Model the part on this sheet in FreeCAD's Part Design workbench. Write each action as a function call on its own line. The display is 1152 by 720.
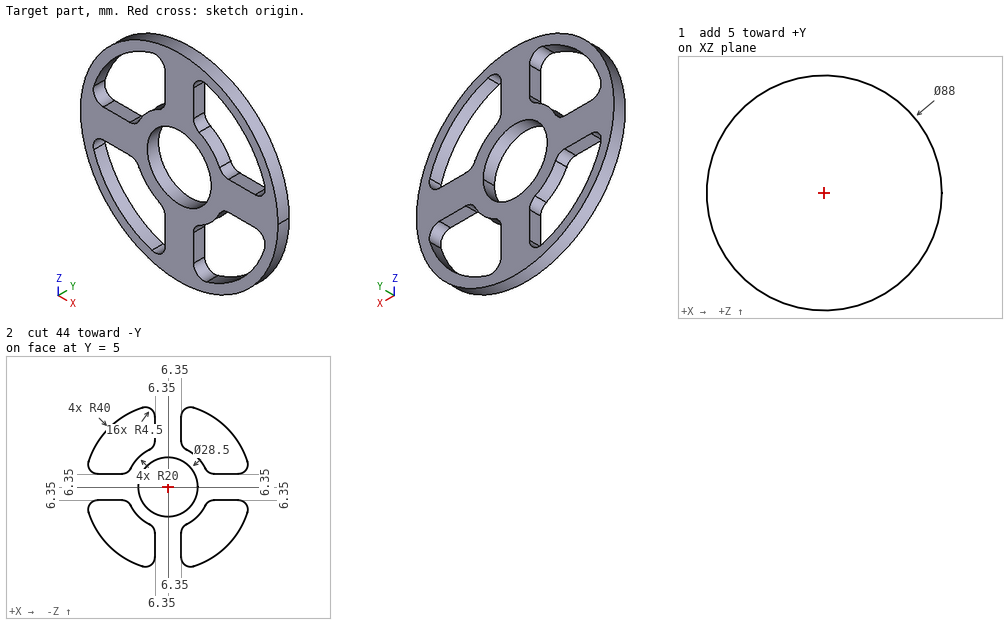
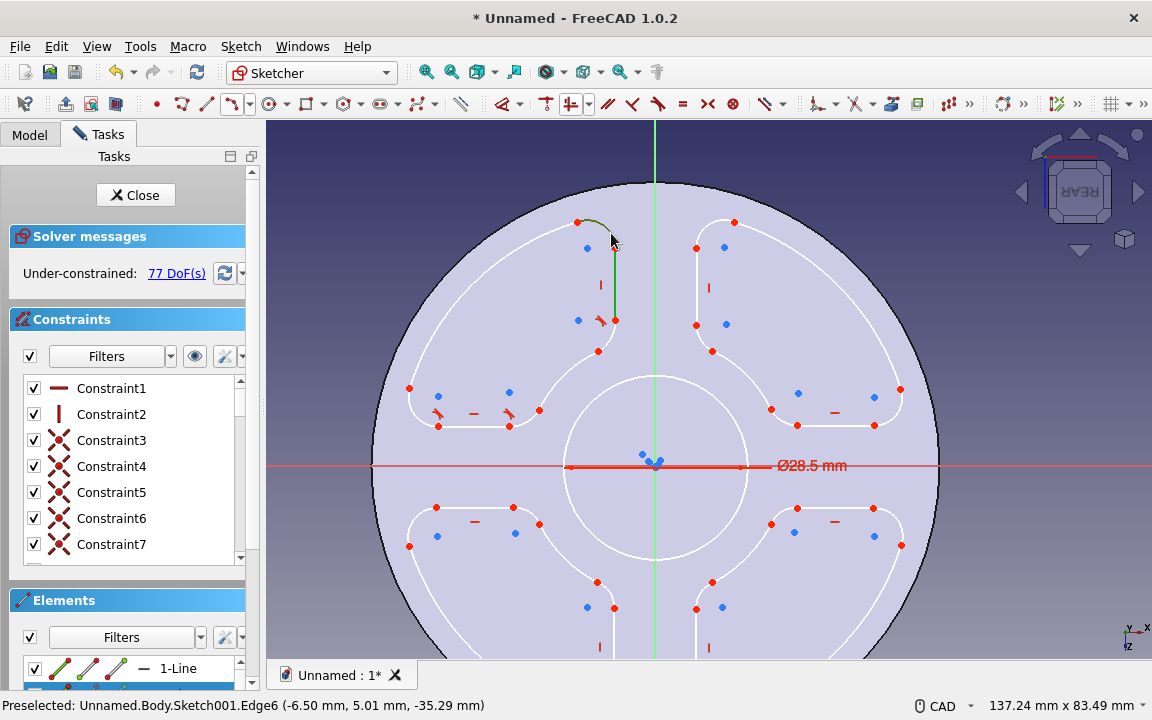
key(t)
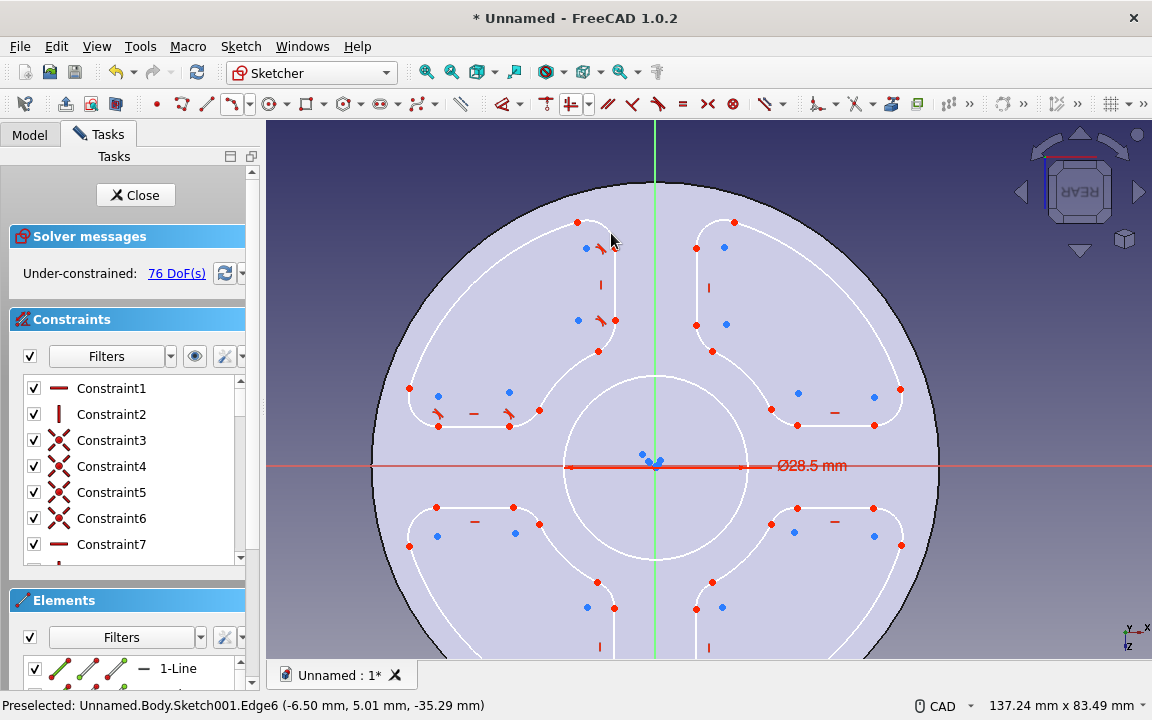
scroll(520, 425, up, 2)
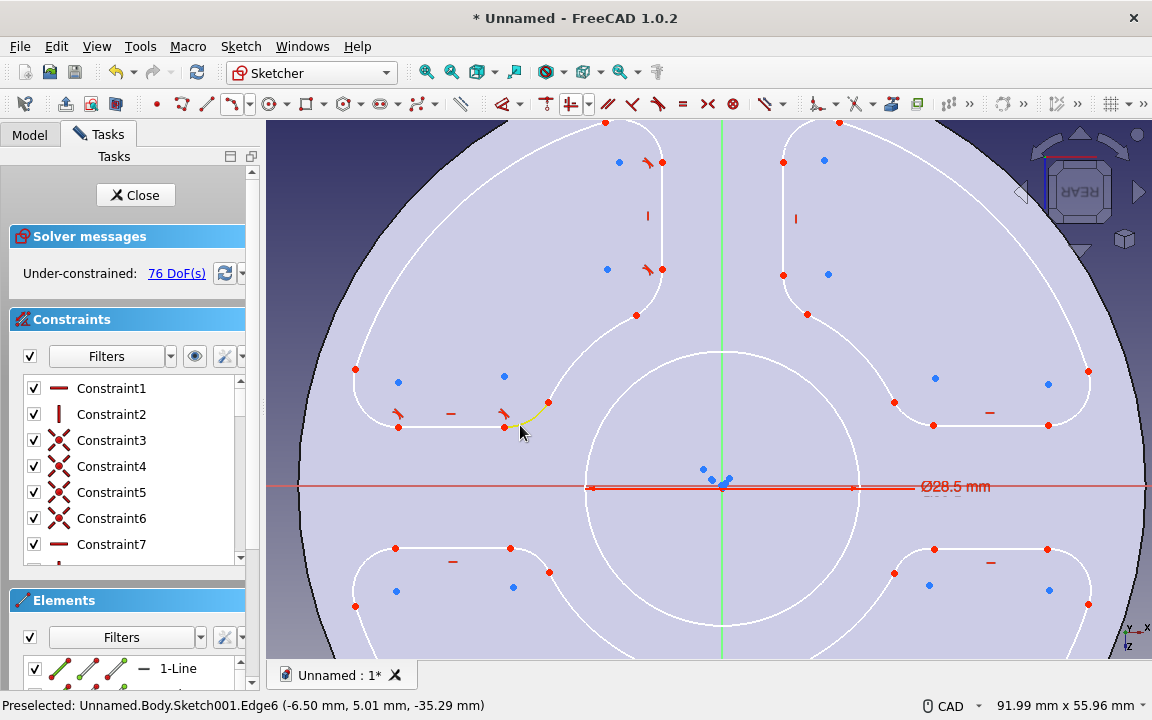
click(520, 425)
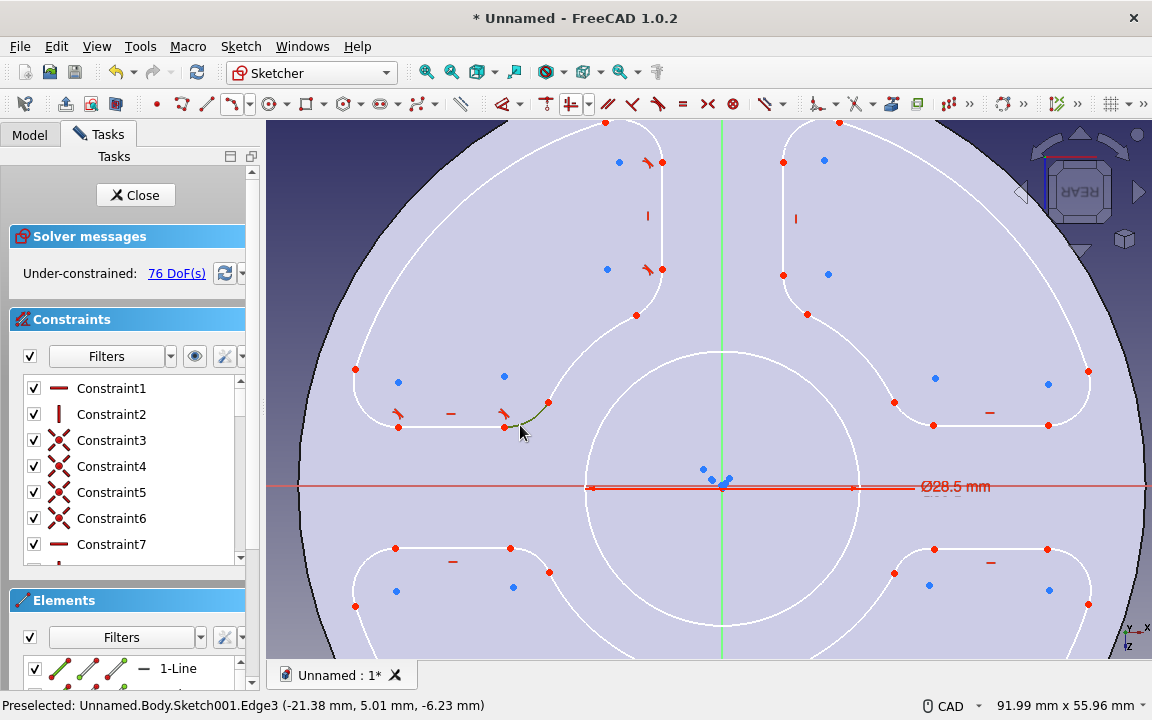
click(604, 335)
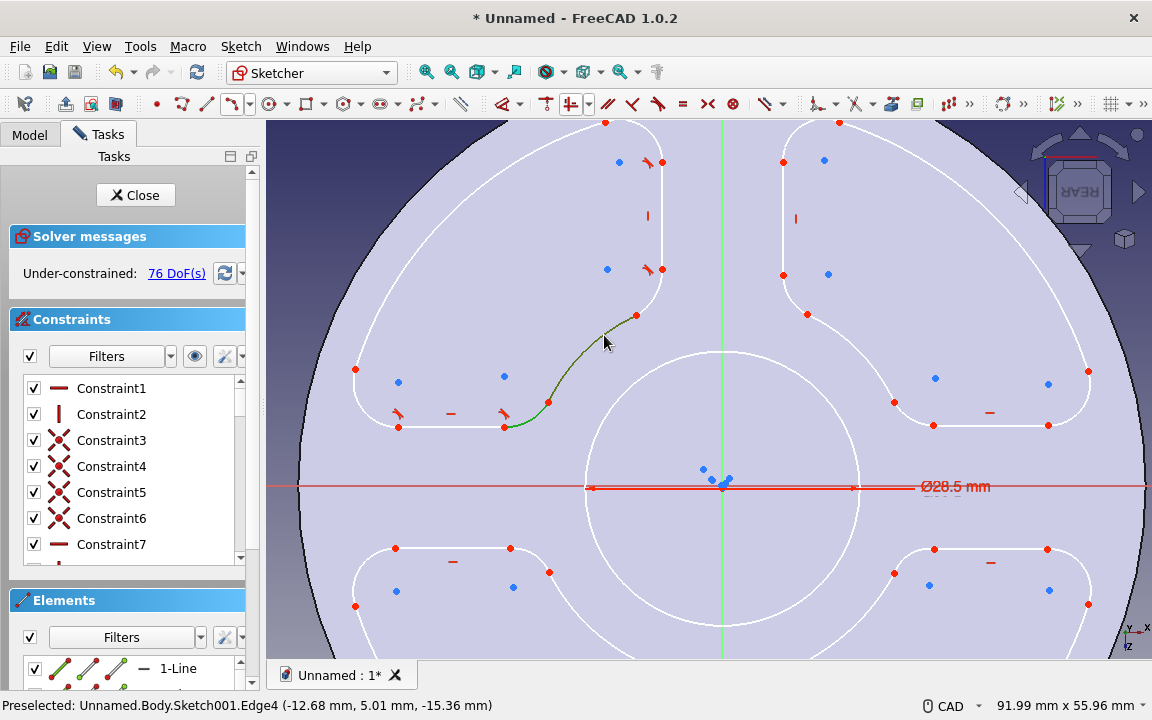
key(t)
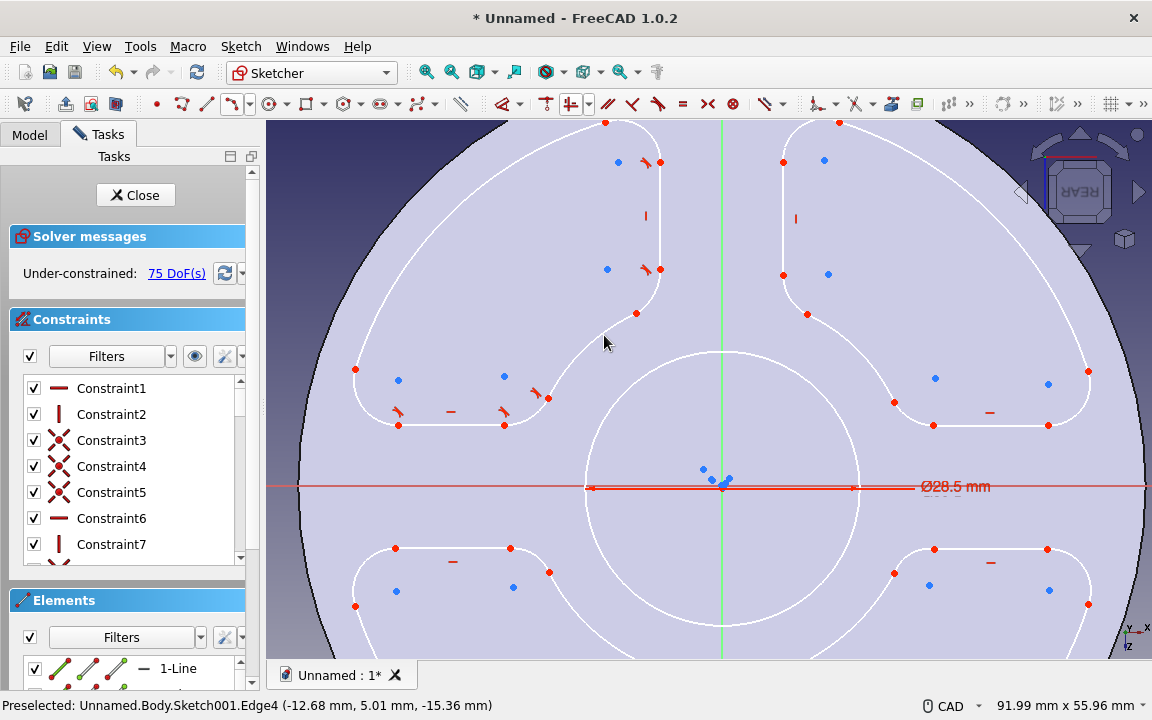
click(604, 332)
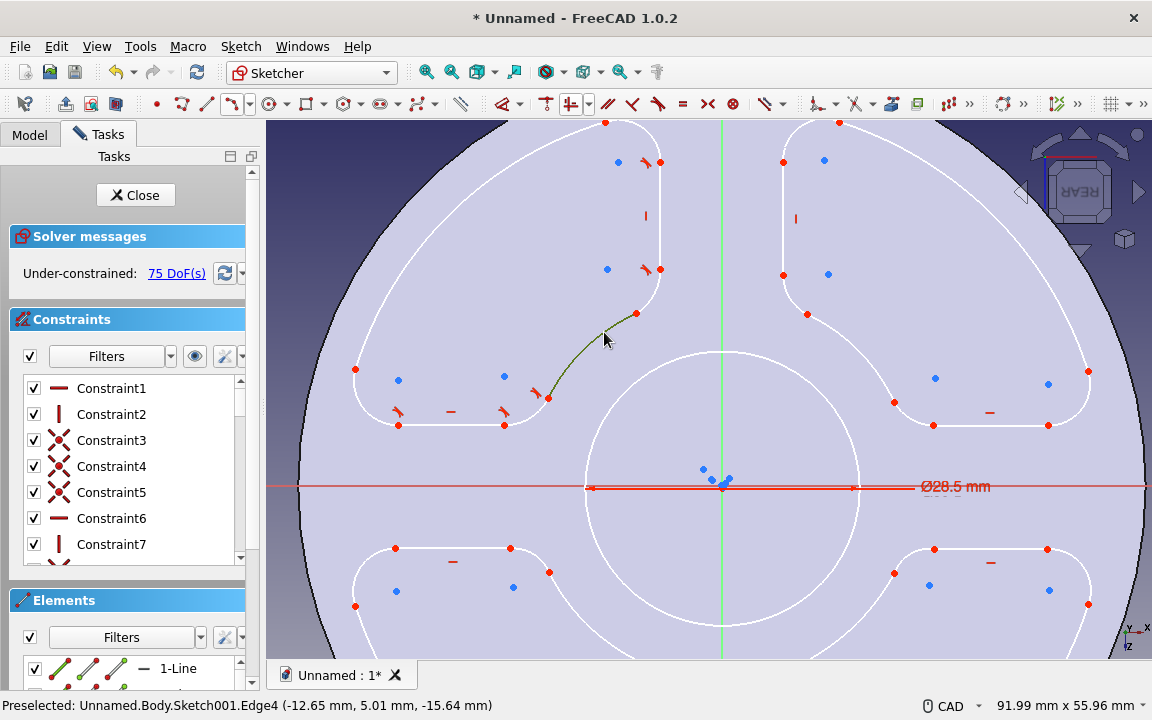
click(648, 303)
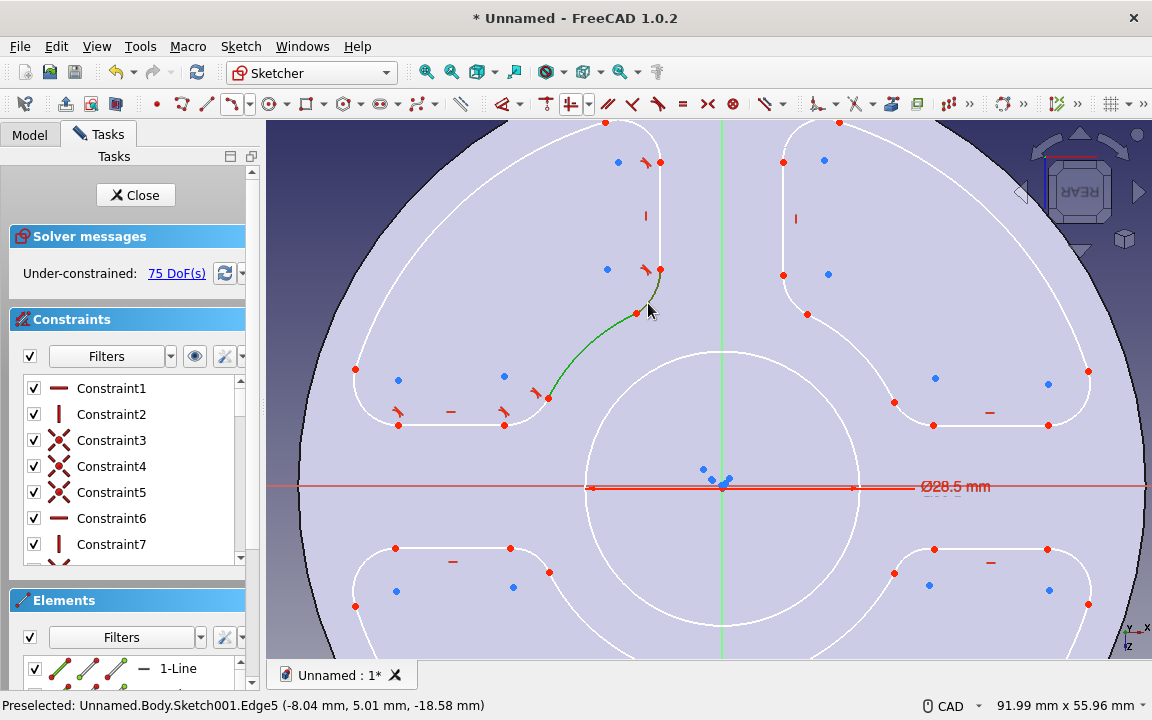
click(658, 104)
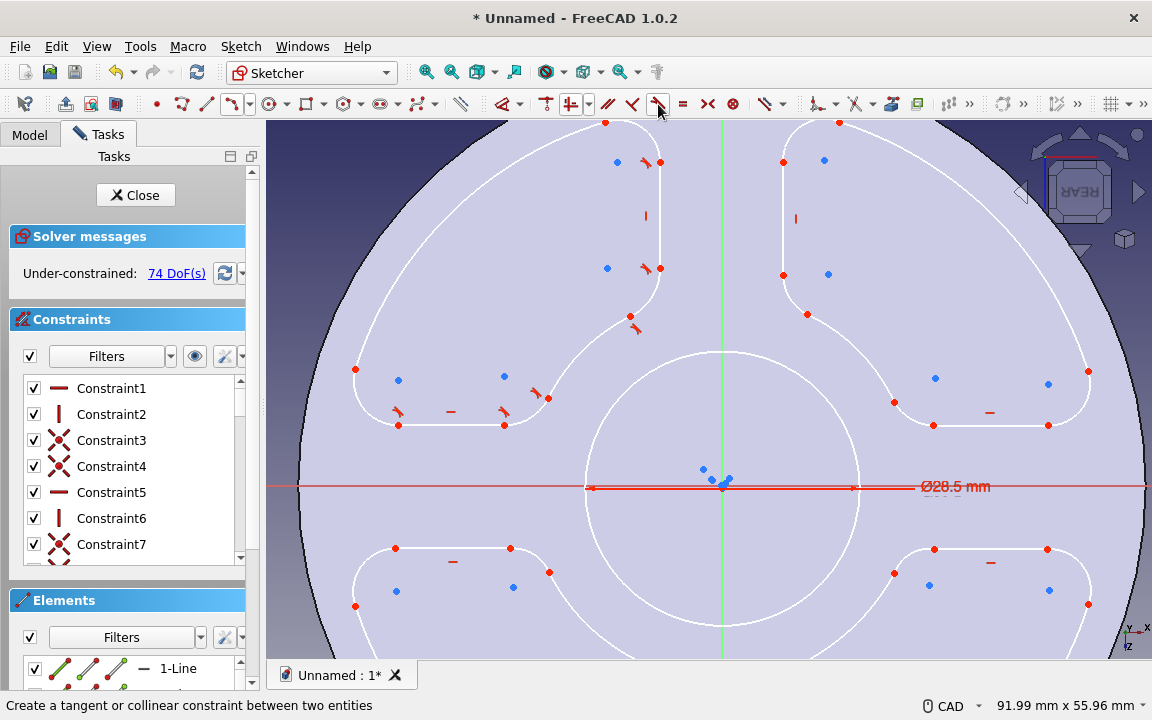
scroll(574, 311, down, 4)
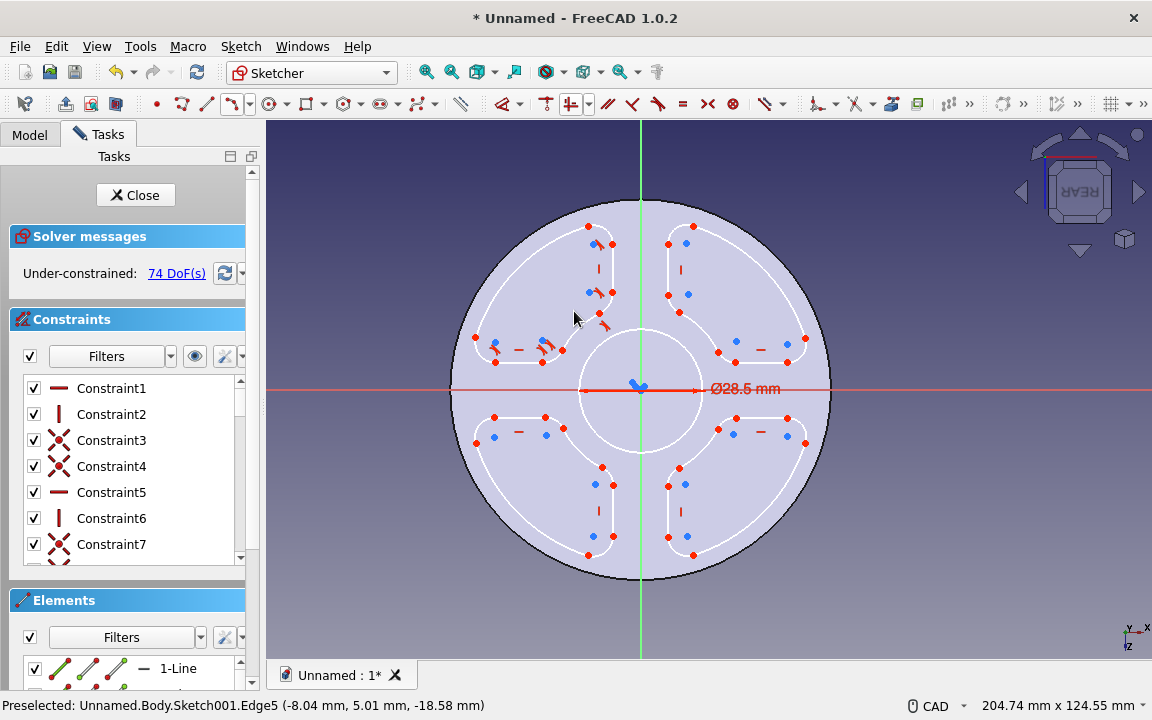
scroll(610, 234, up, 2)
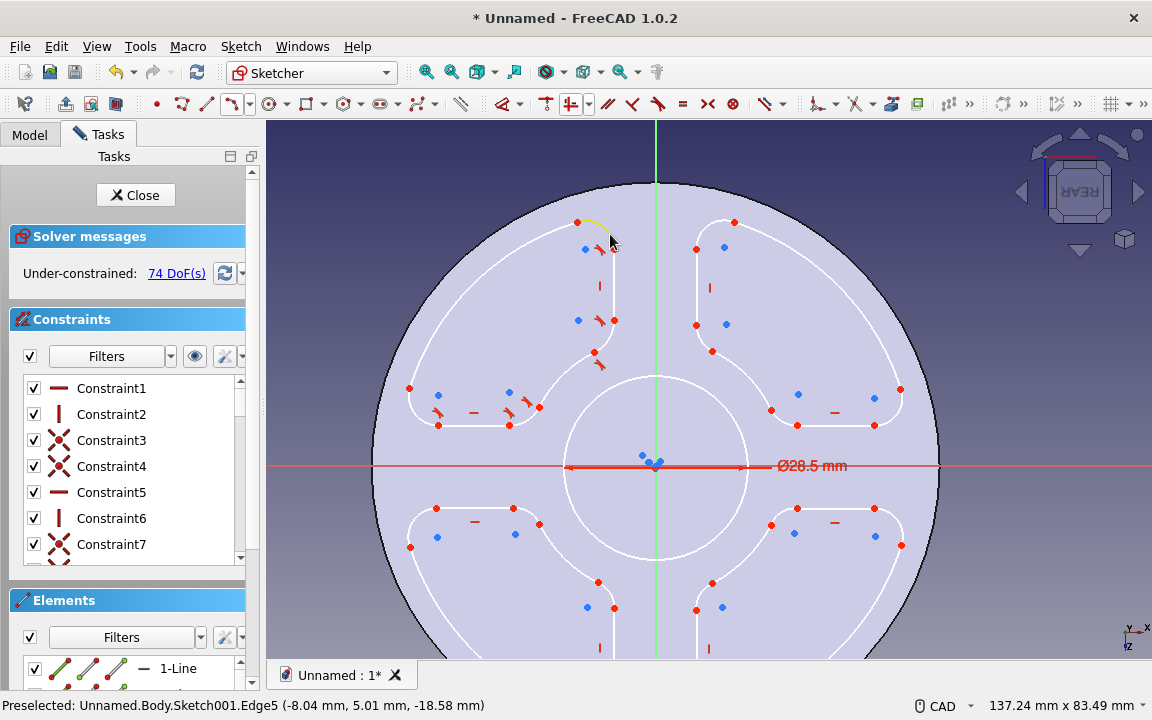
click(610, 234)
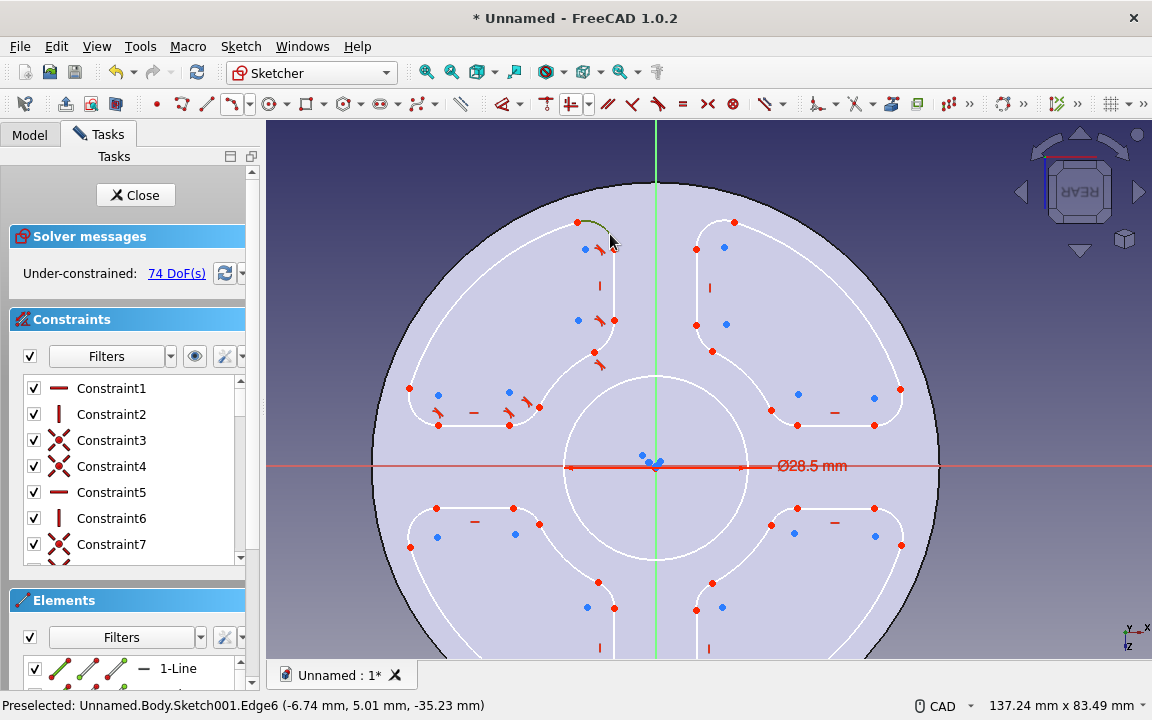
click(511, 254)